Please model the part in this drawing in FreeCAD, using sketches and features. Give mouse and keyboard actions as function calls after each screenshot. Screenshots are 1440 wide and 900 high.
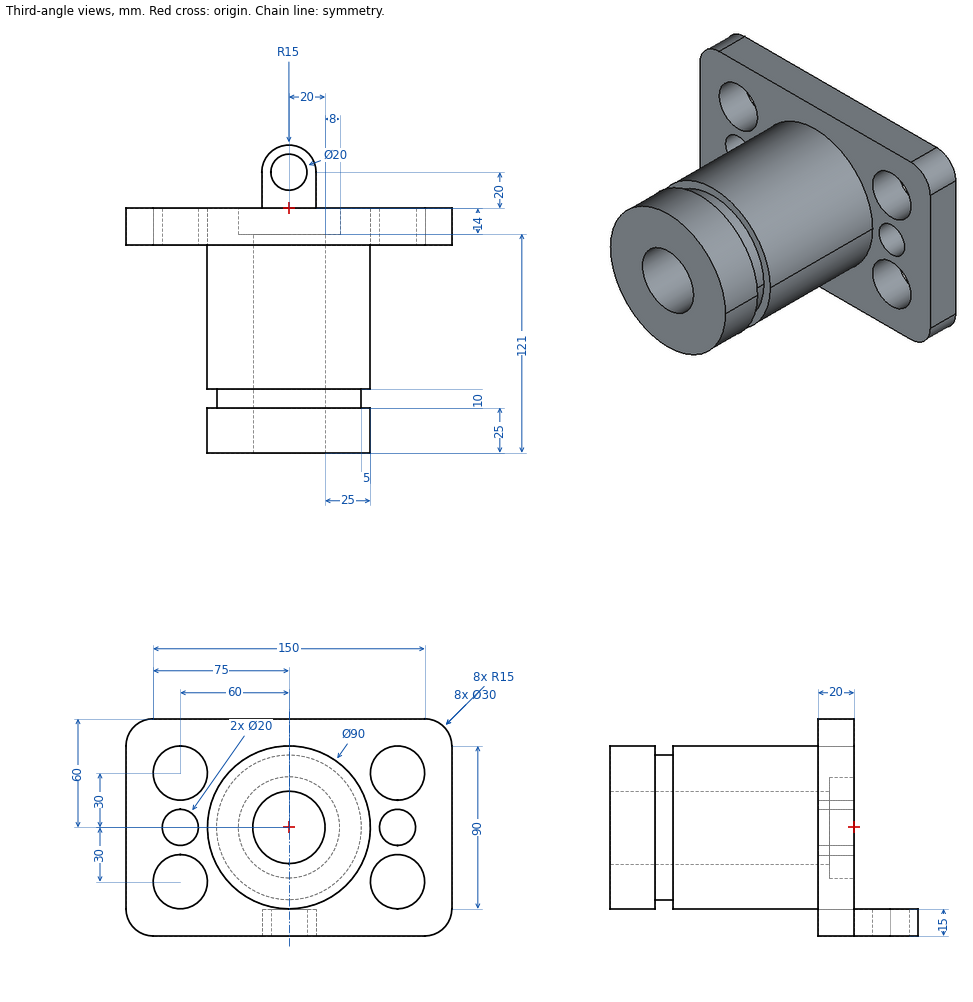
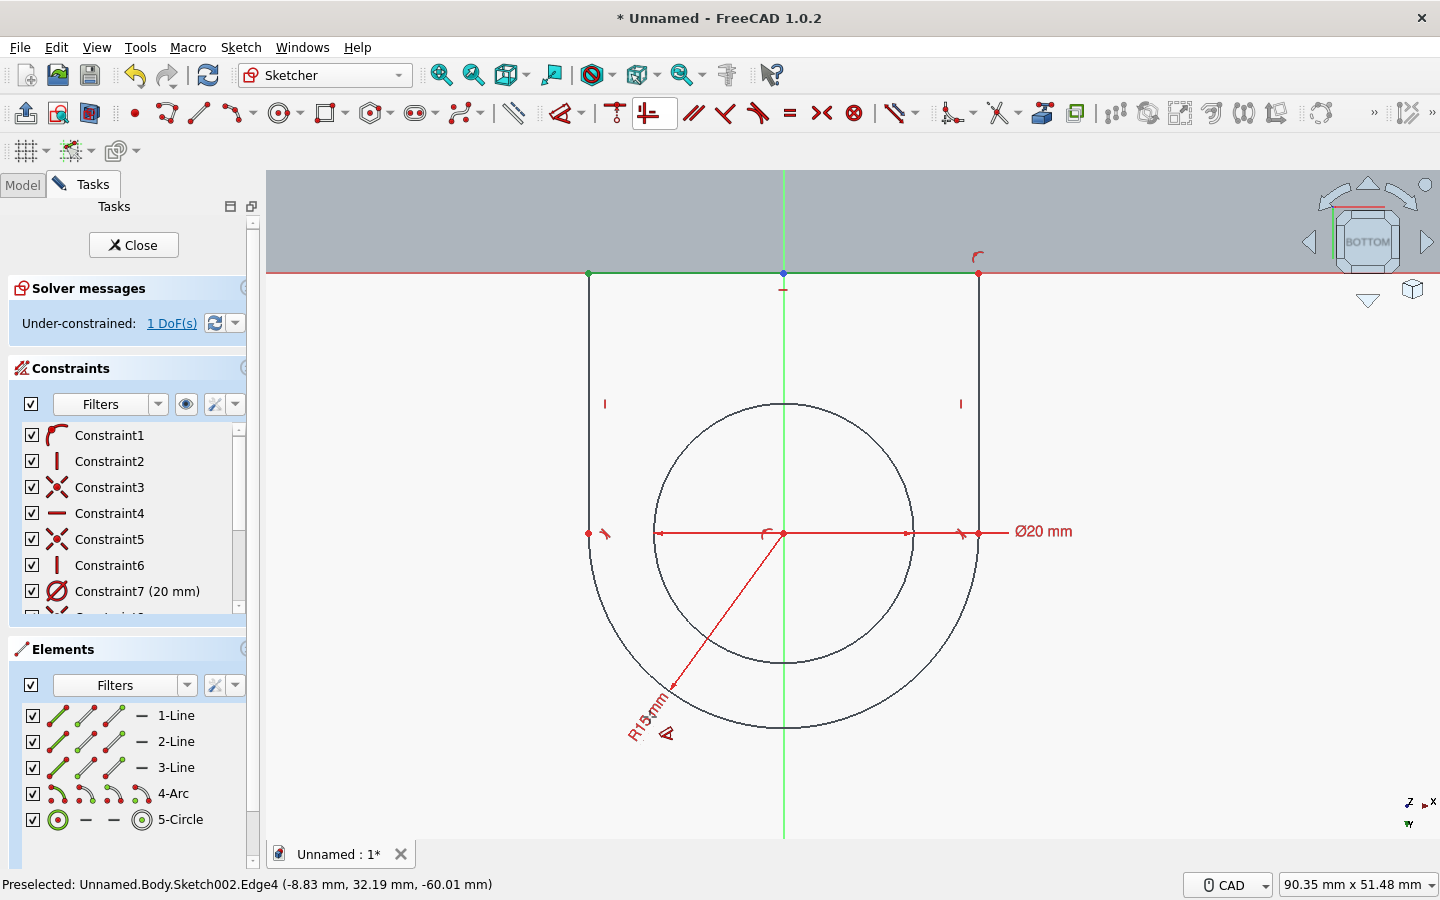
click(979, 455)
click(1013, 403)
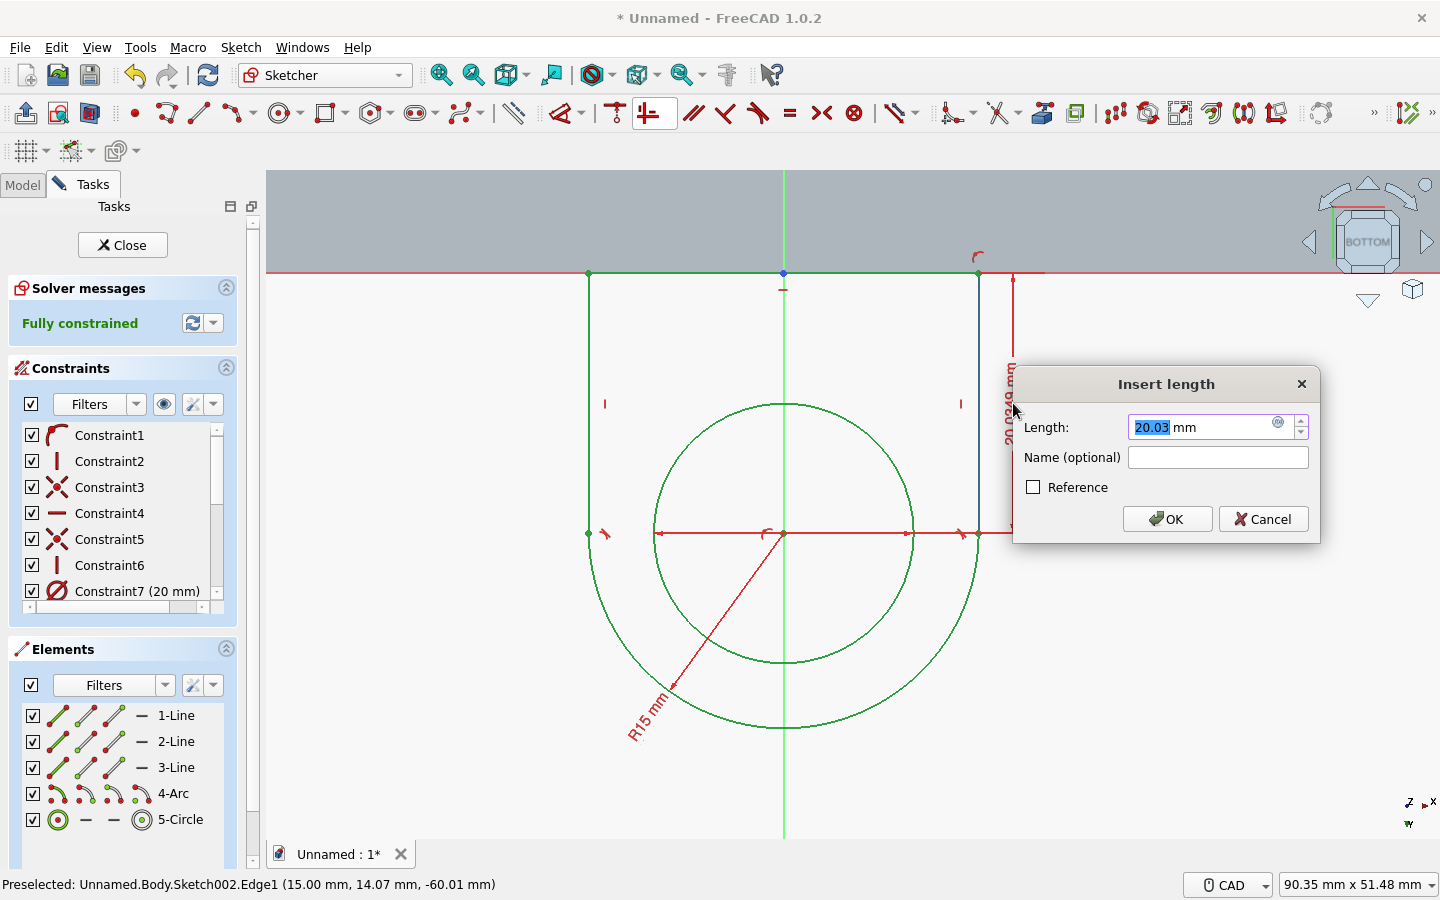
text(20)
key(Return)
key(Escape)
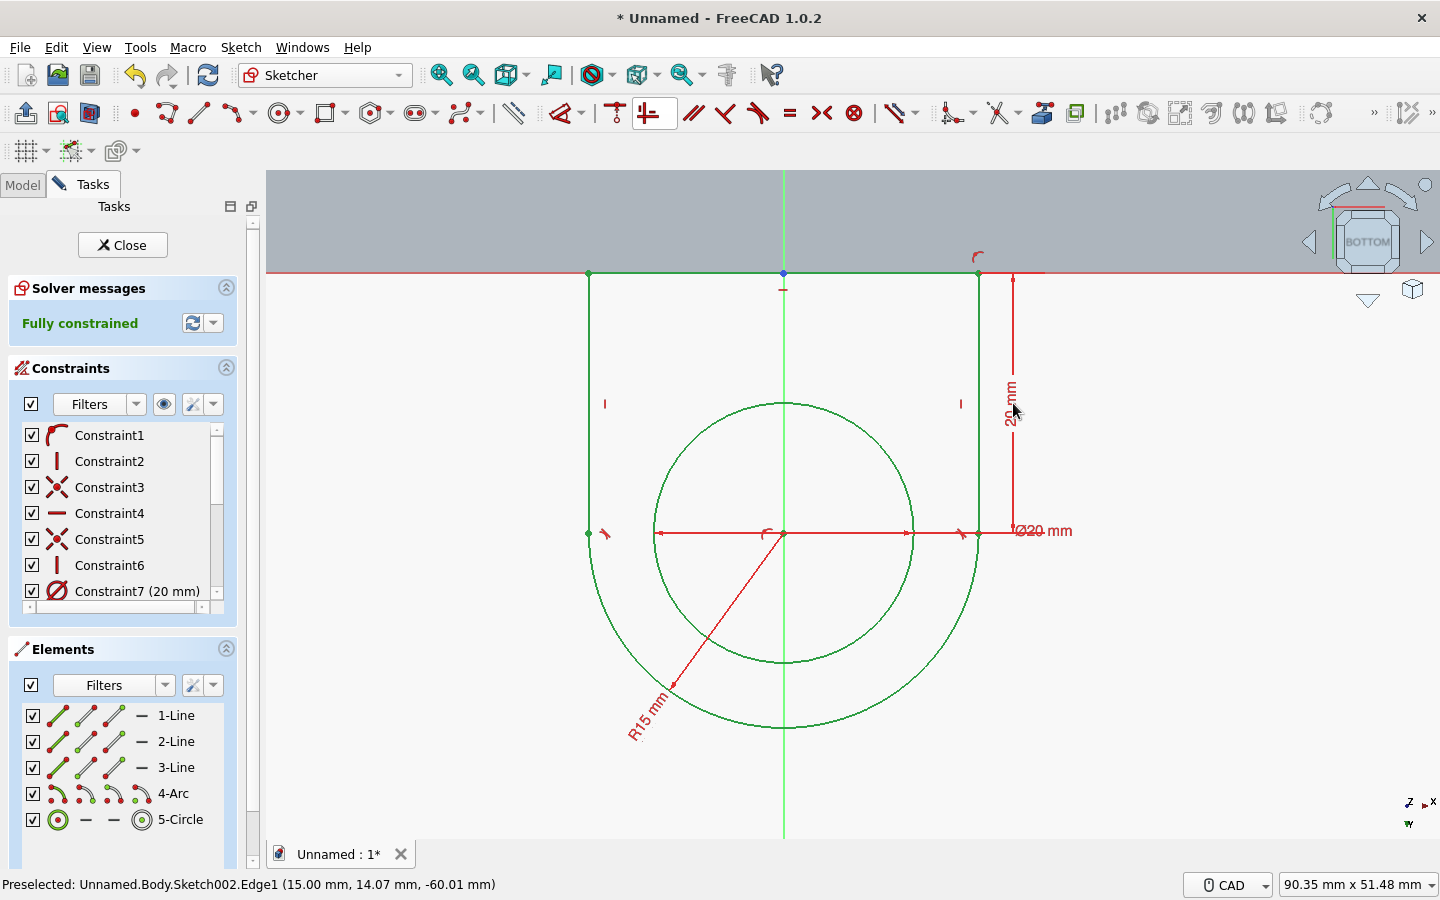
click(123, 245)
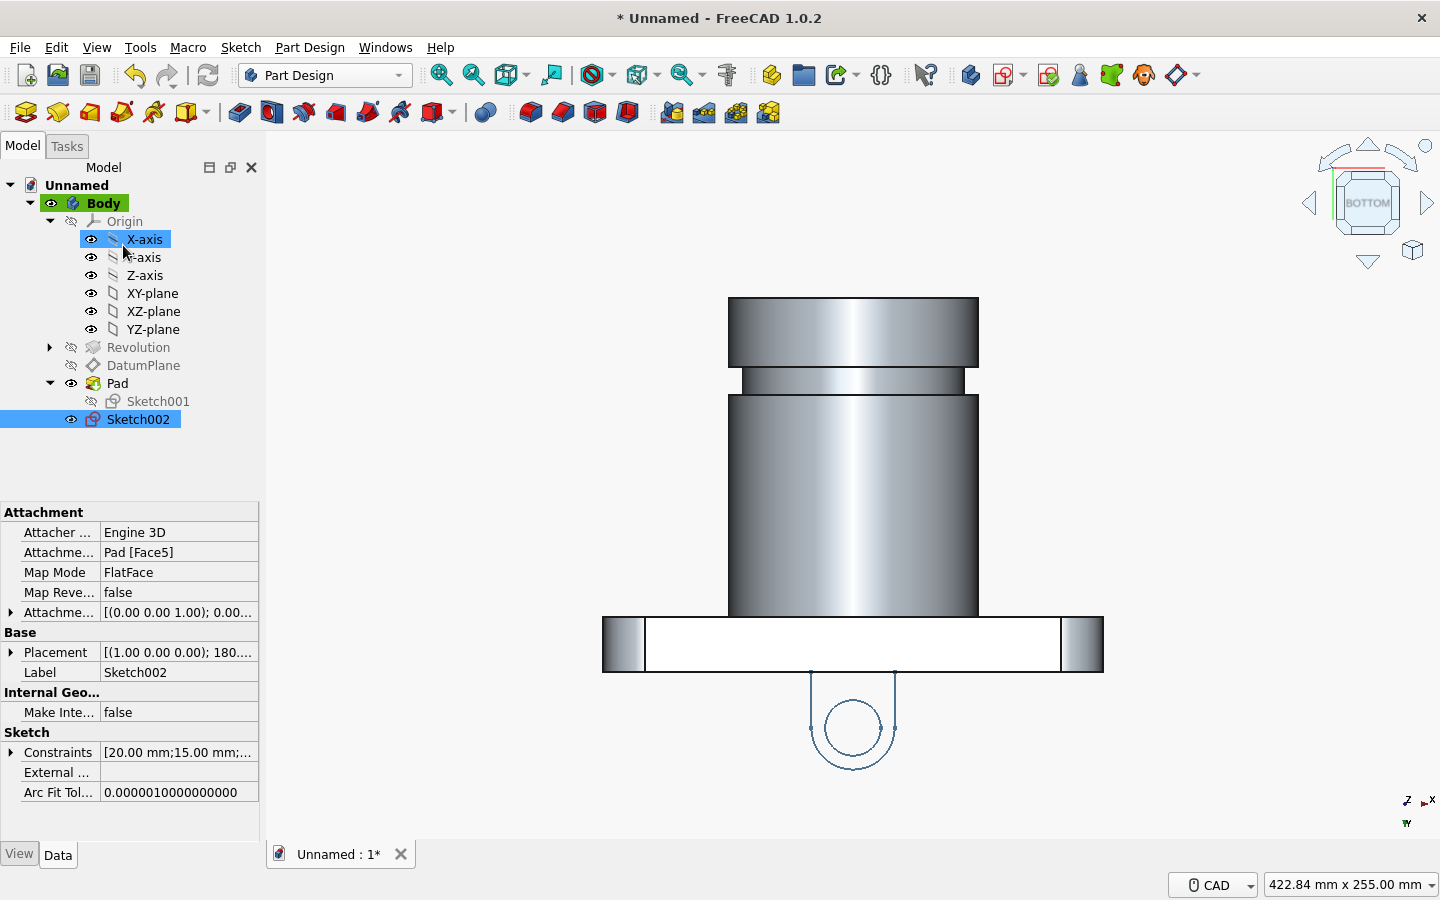
click(26, 112)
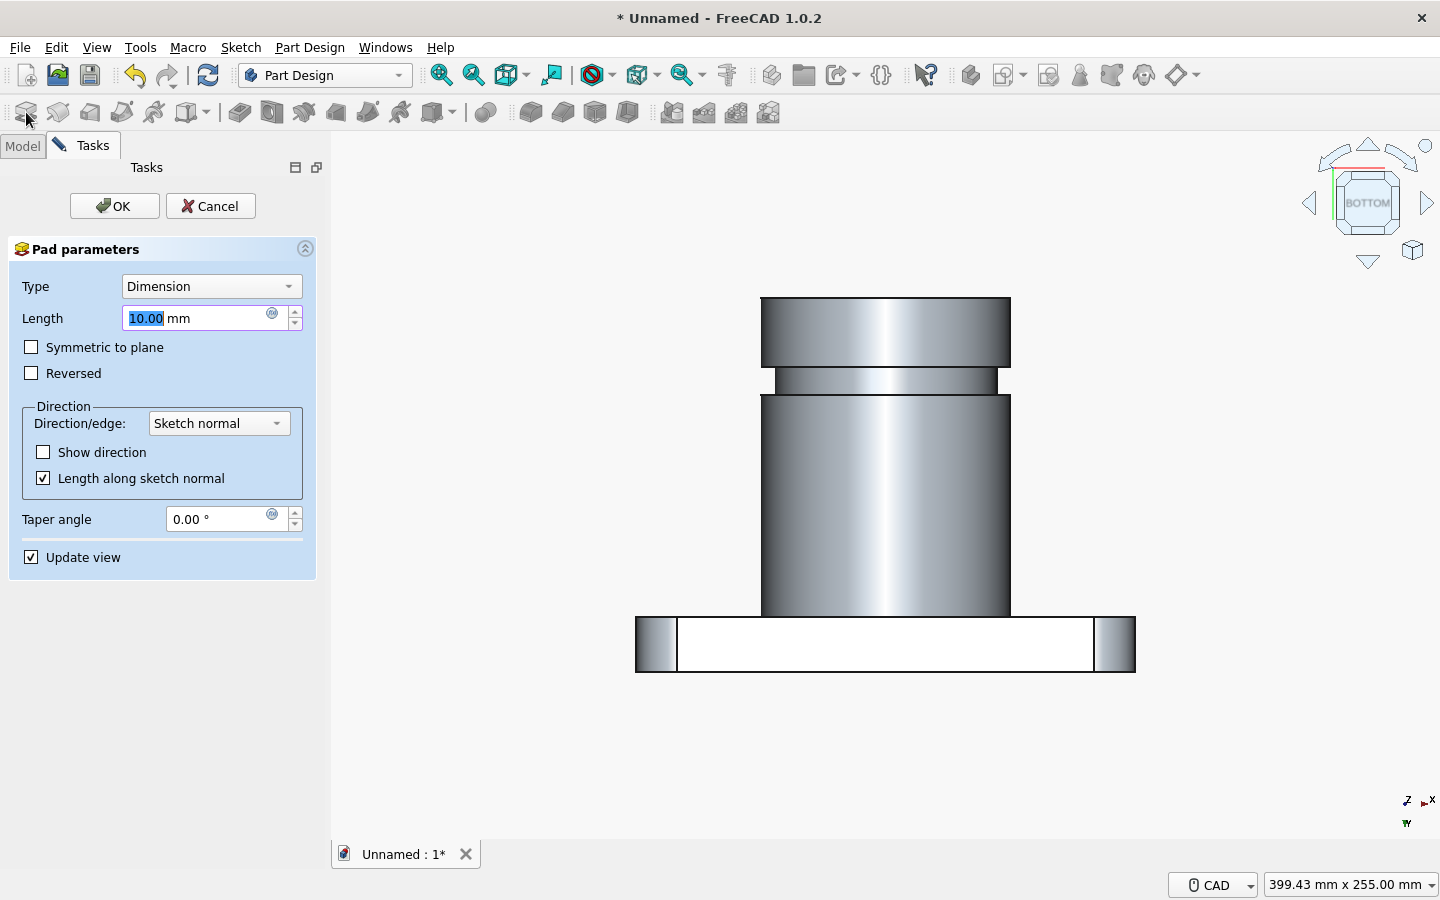
text(15)
key(Tab)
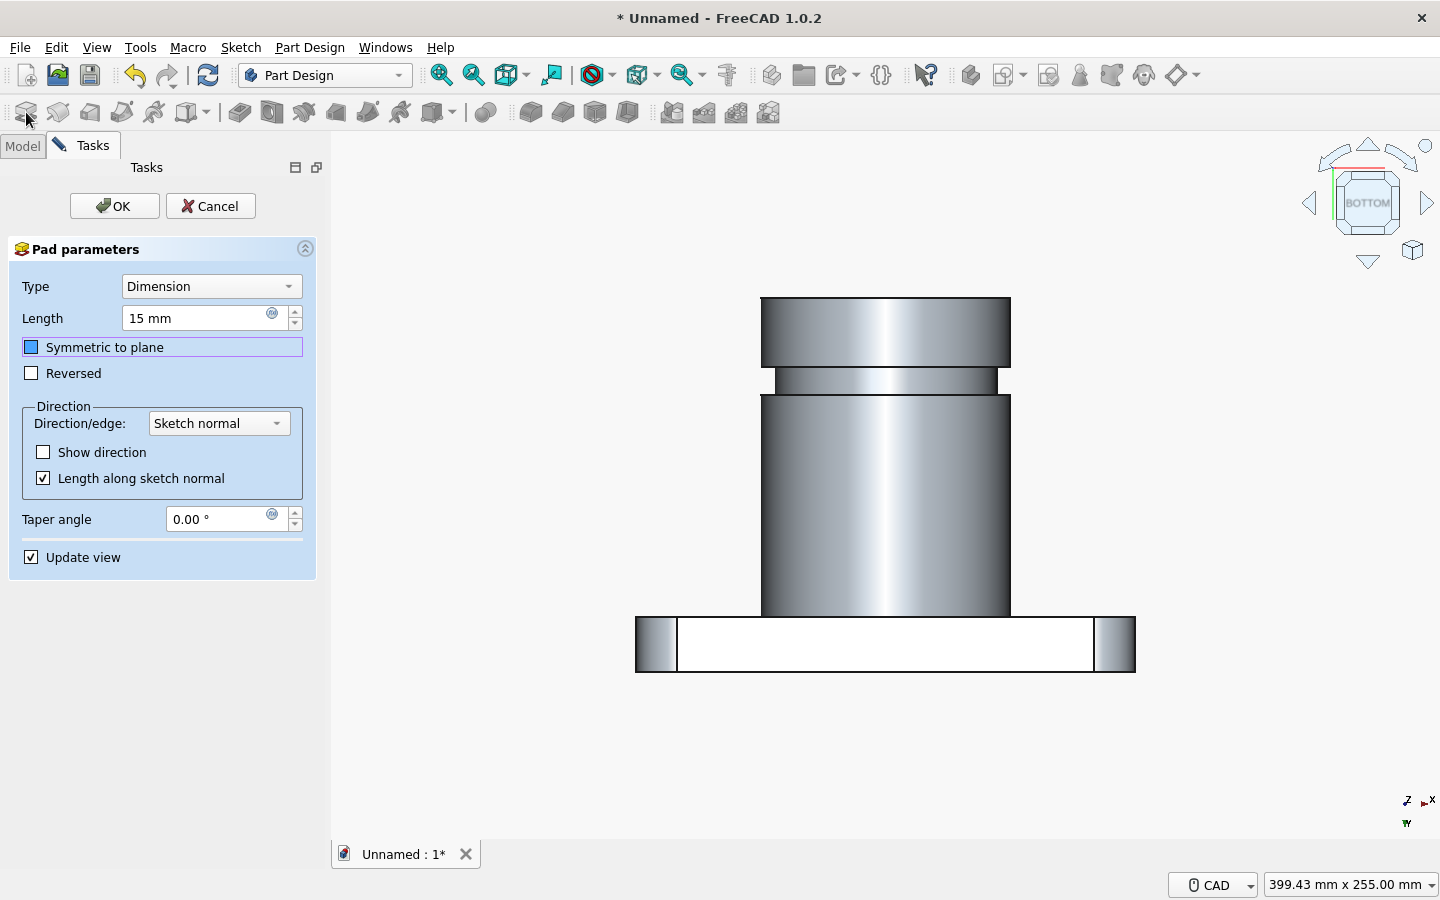
click(30, 373)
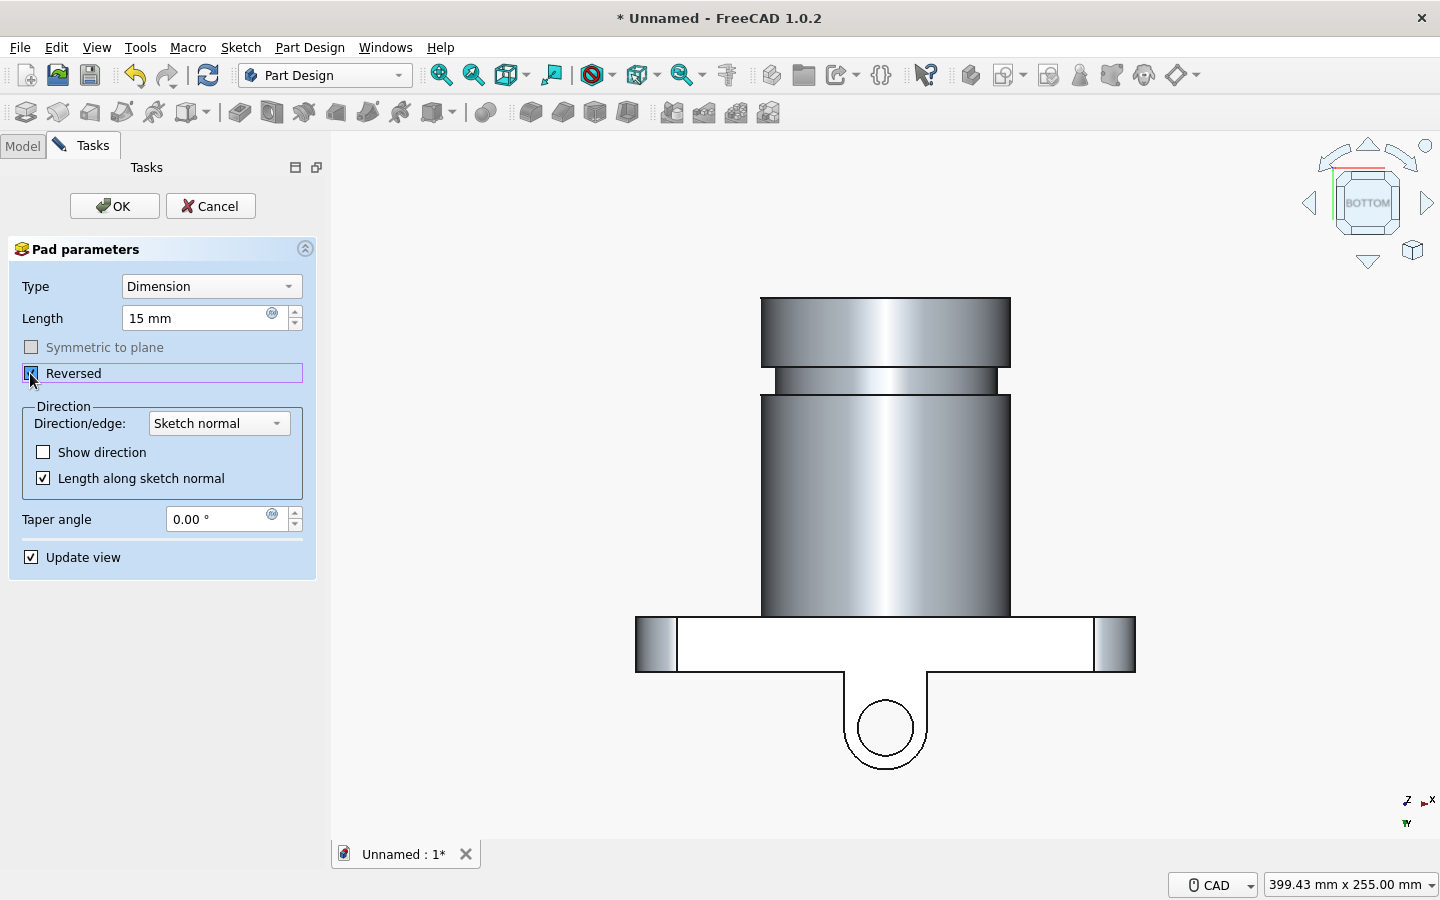
click(115, 206)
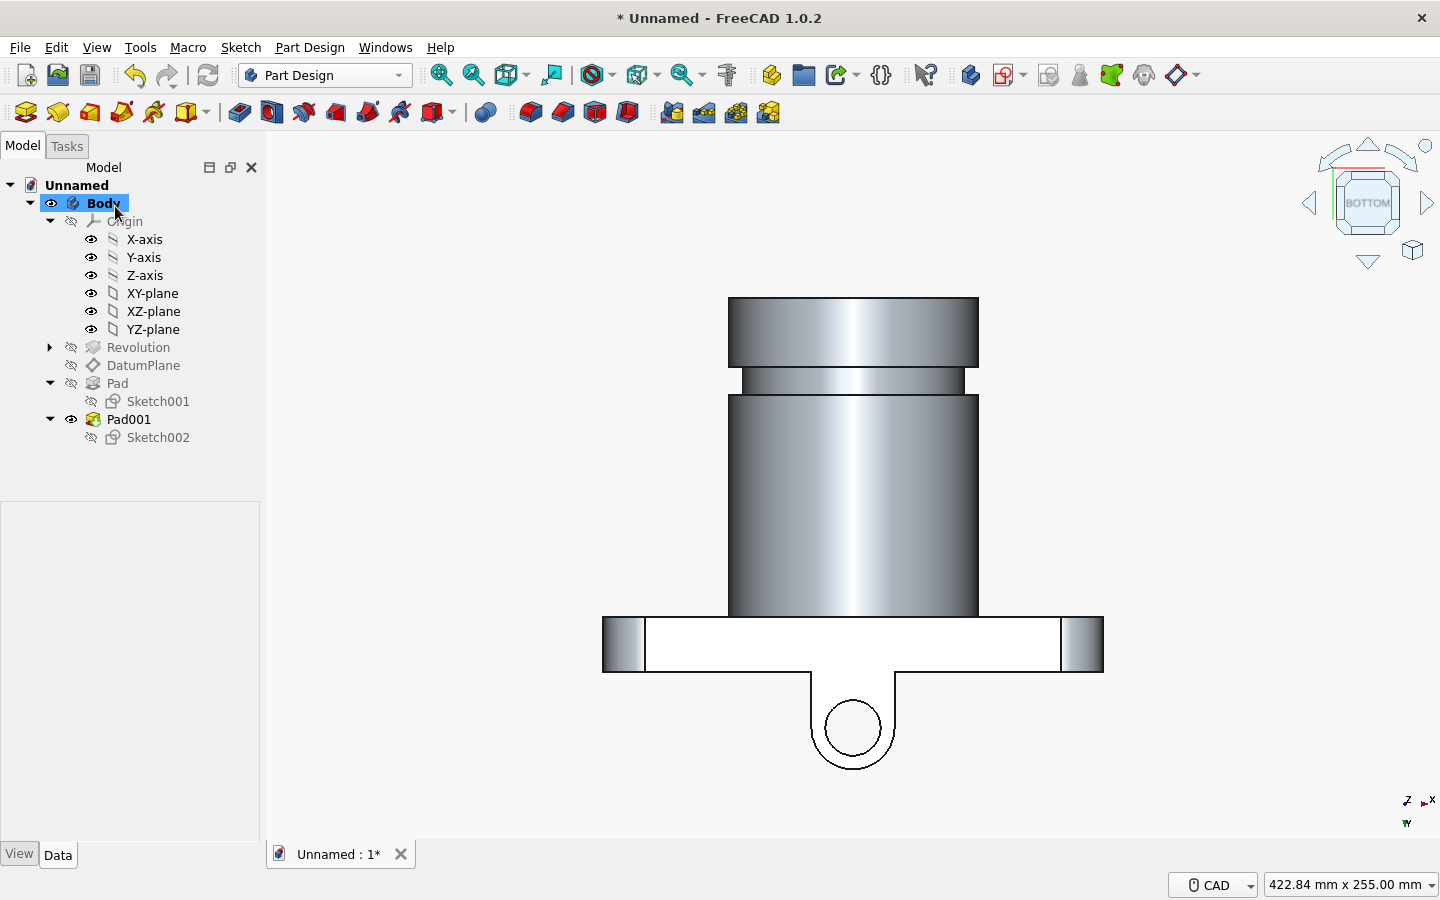
key(0)